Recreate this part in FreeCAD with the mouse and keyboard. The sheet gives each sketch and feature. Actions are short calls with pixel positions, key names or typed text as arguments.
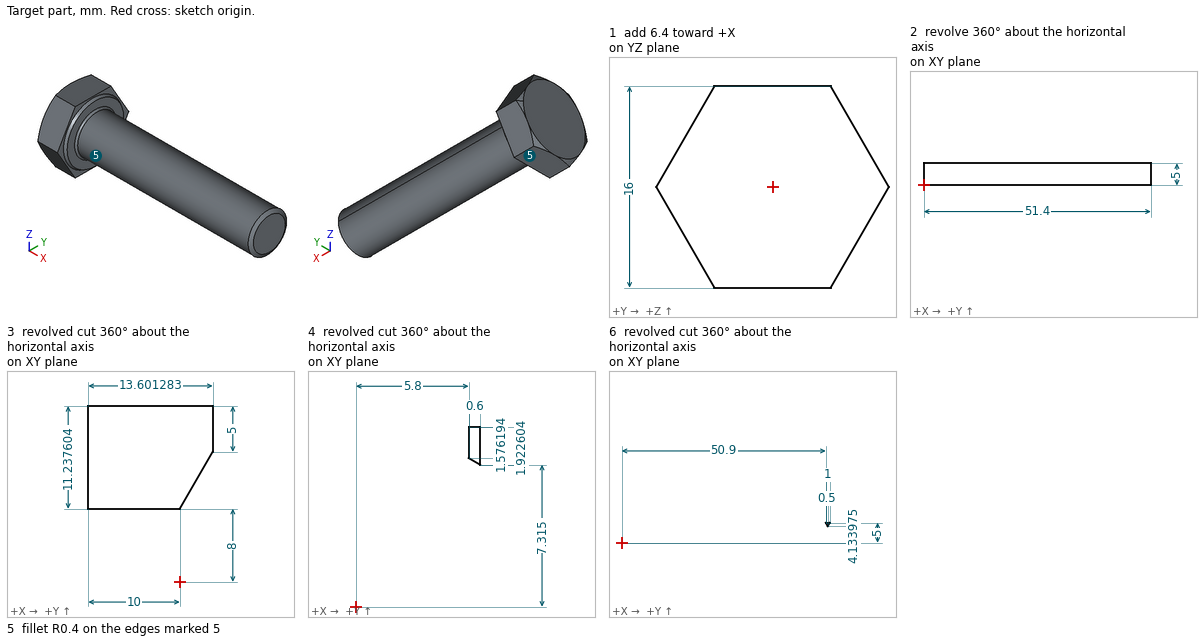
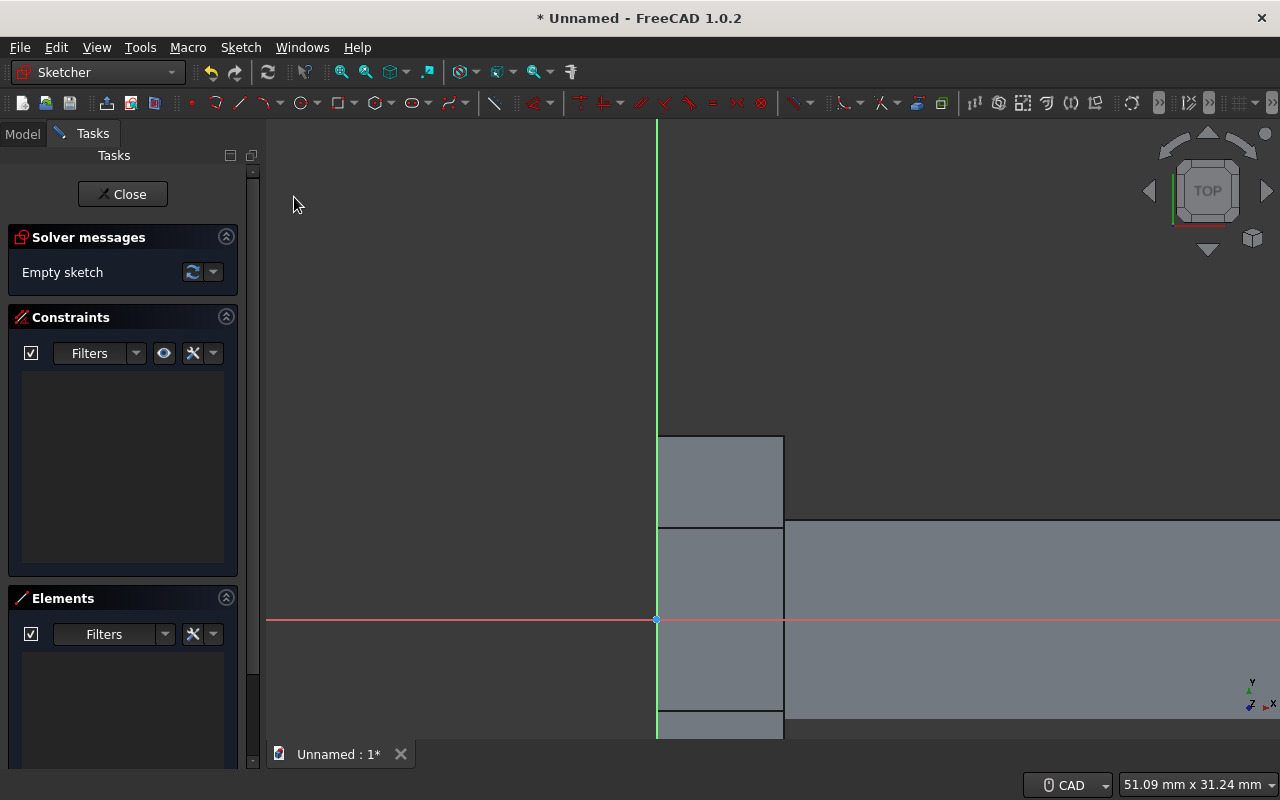
click(216, 104)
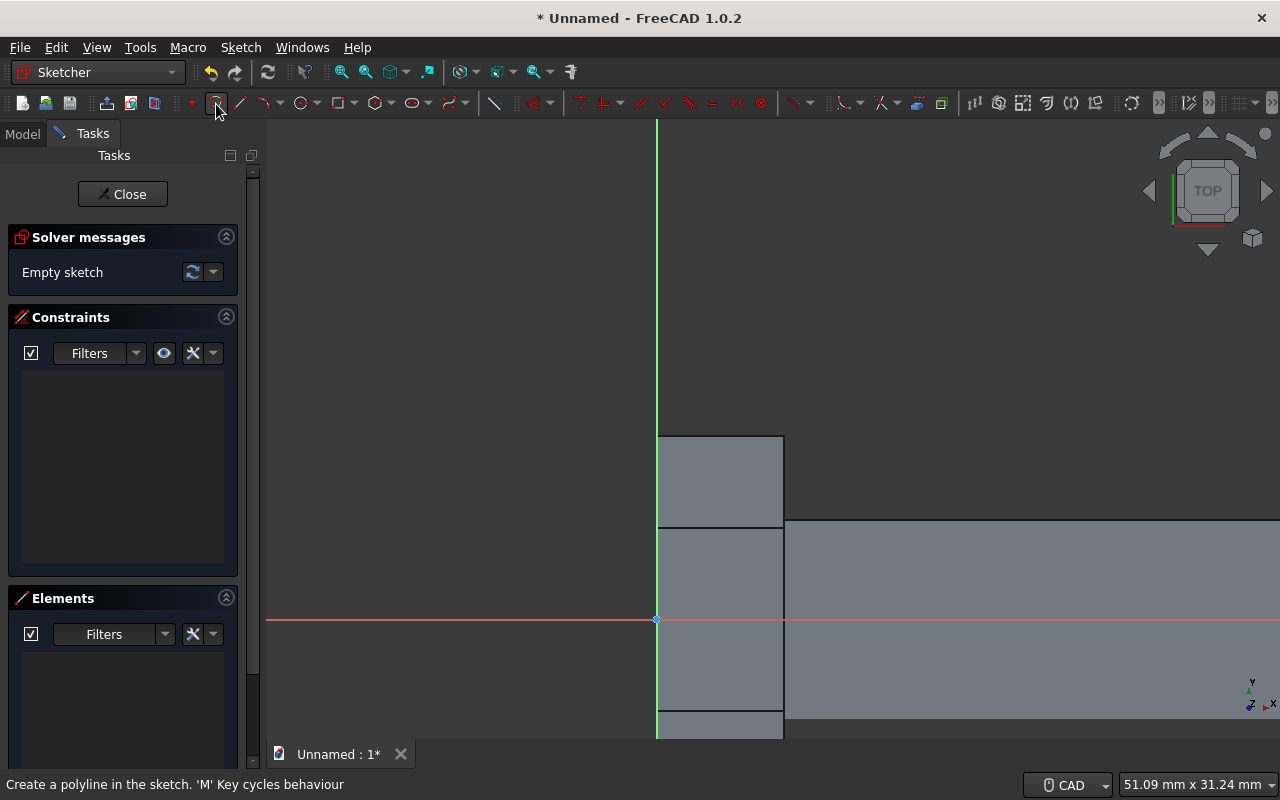
click(657, 461)
click(728, 337)
click(728, 238)
click(458, 238)
click(458, 461)
click(657, 462)
key(Escape)
key(Escape)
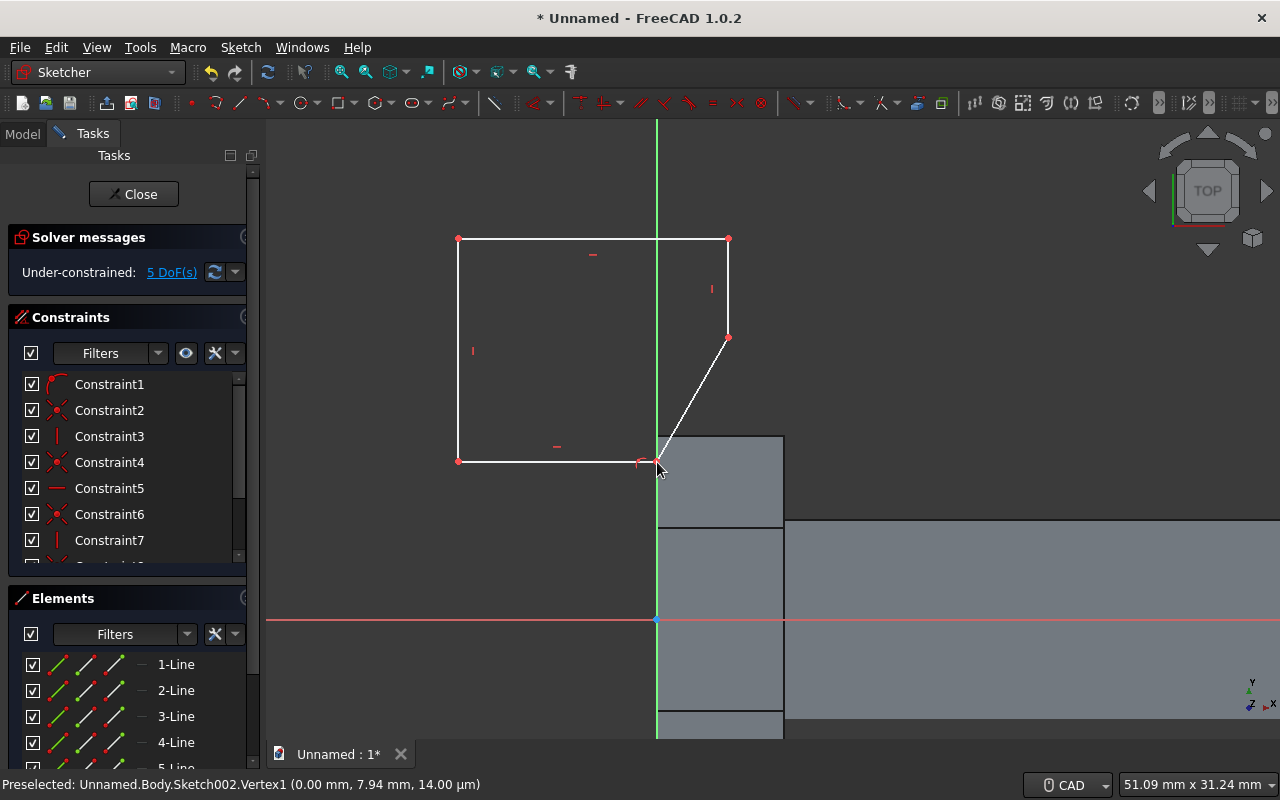
click(534, 104)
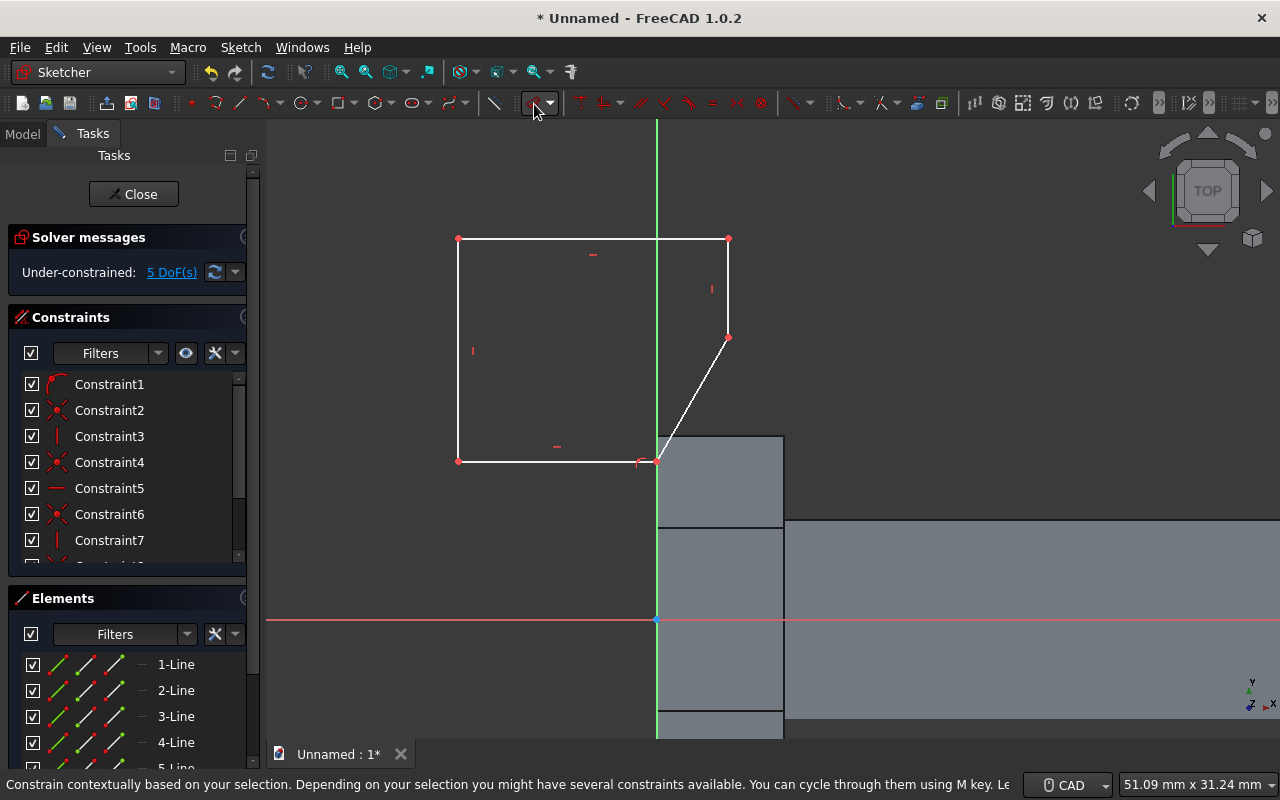
click(728, 308)
click(762, 288)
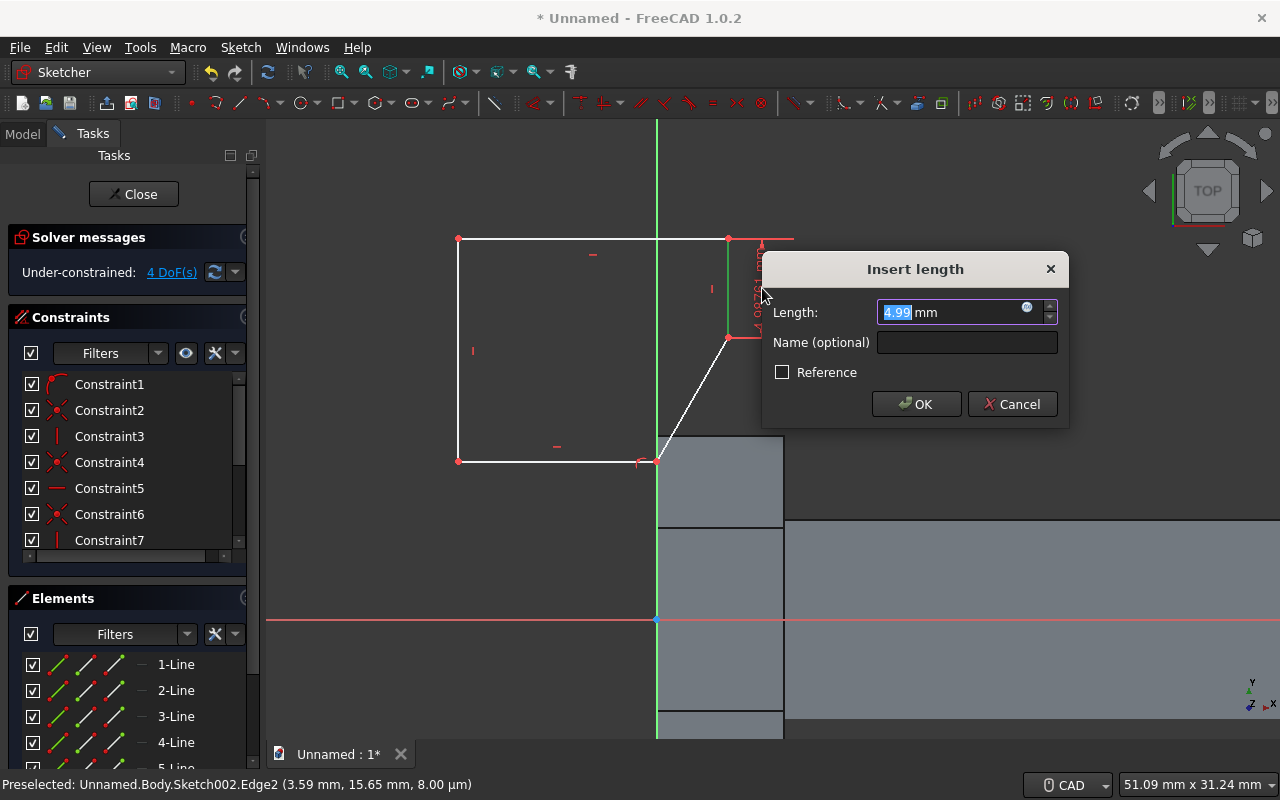
text(5)
key(Return)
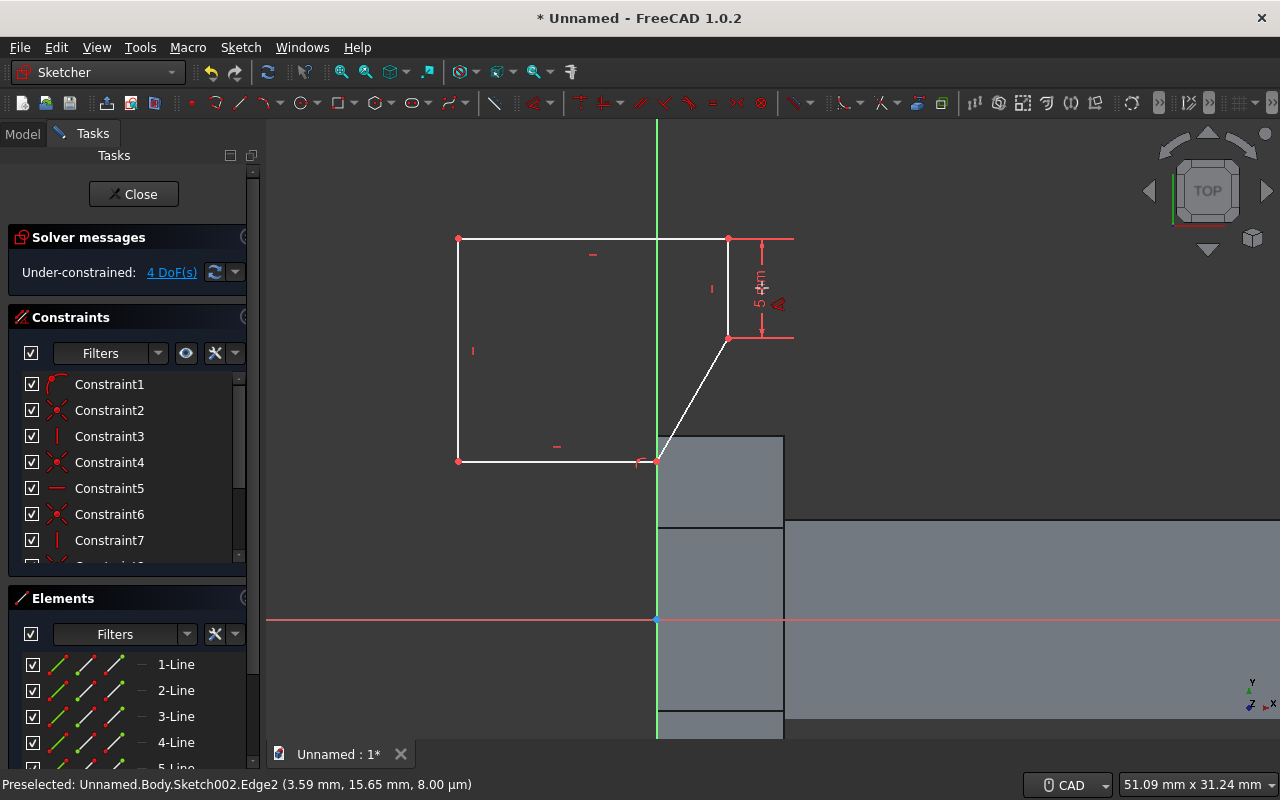
click(518, 462)
click(557, 496)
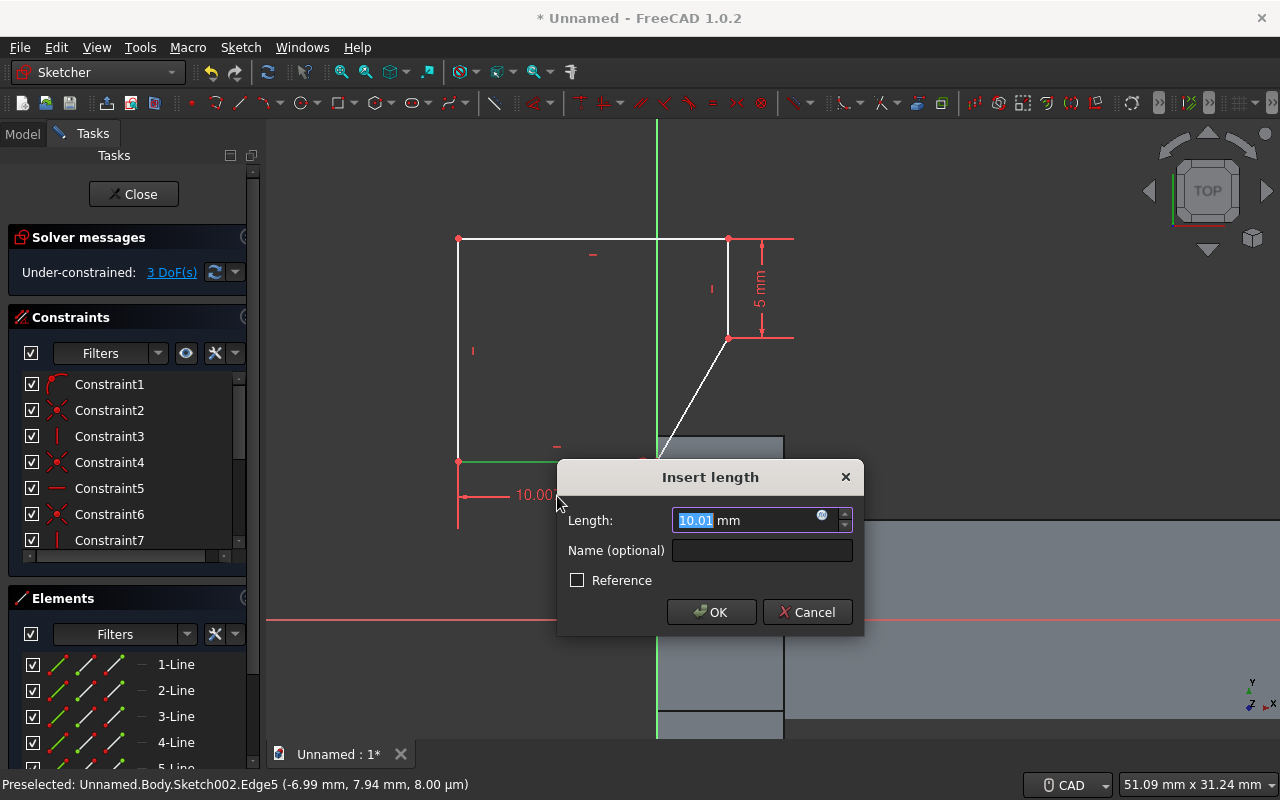
text(10)
key(Return)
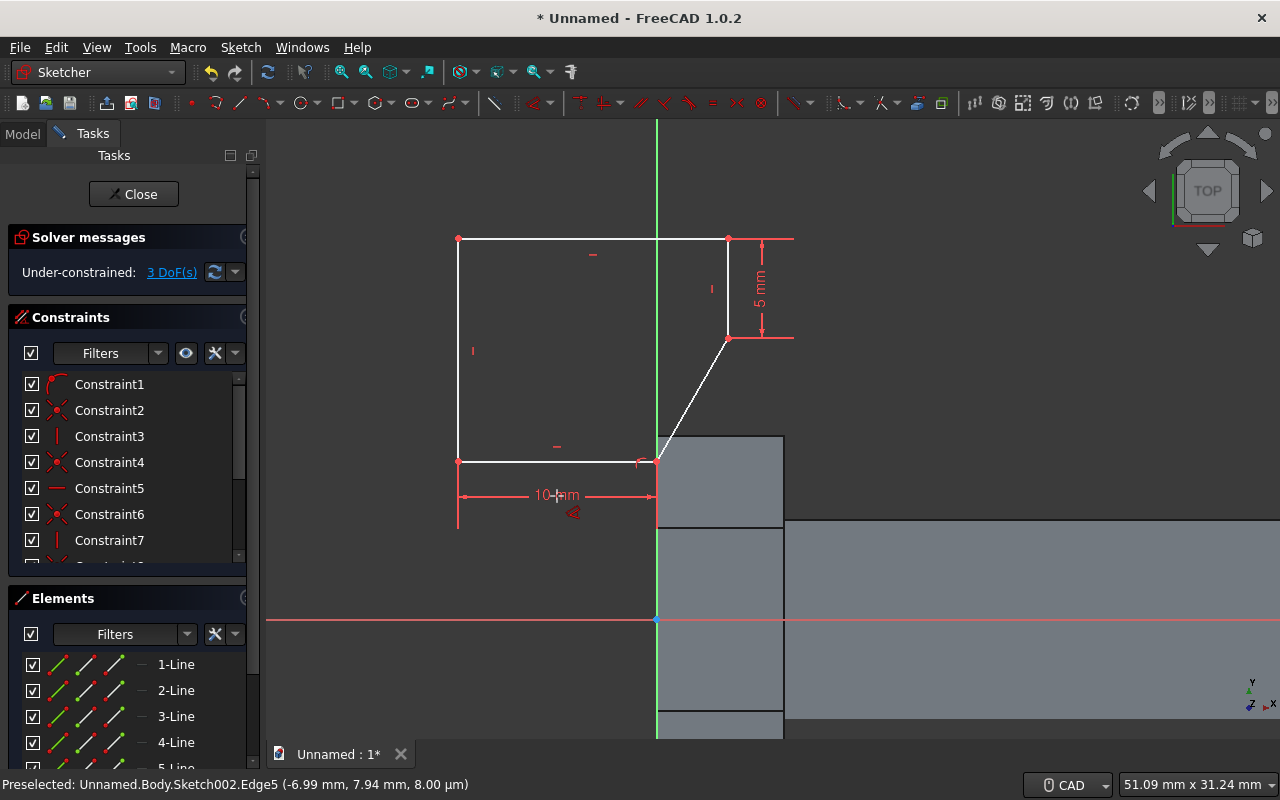
click(657, 462)
click(691, 541)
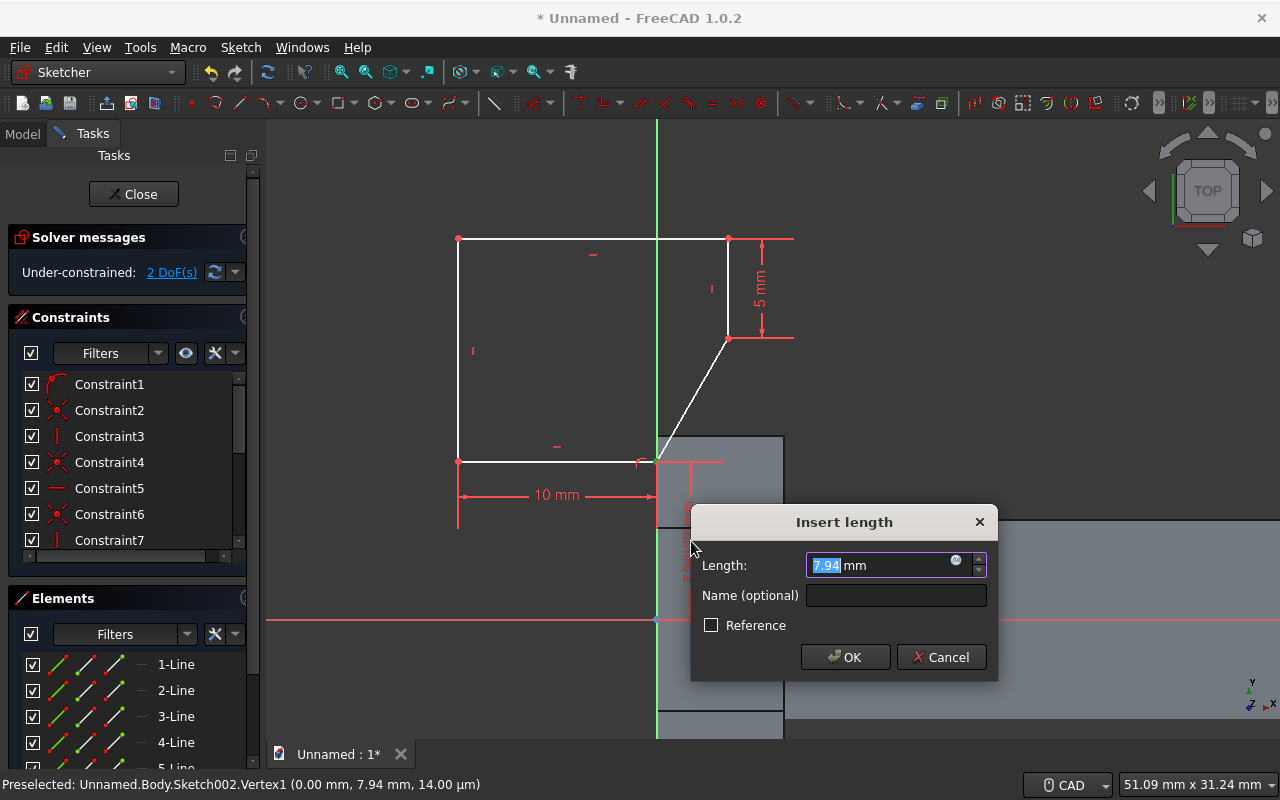
text(8)
key(Return)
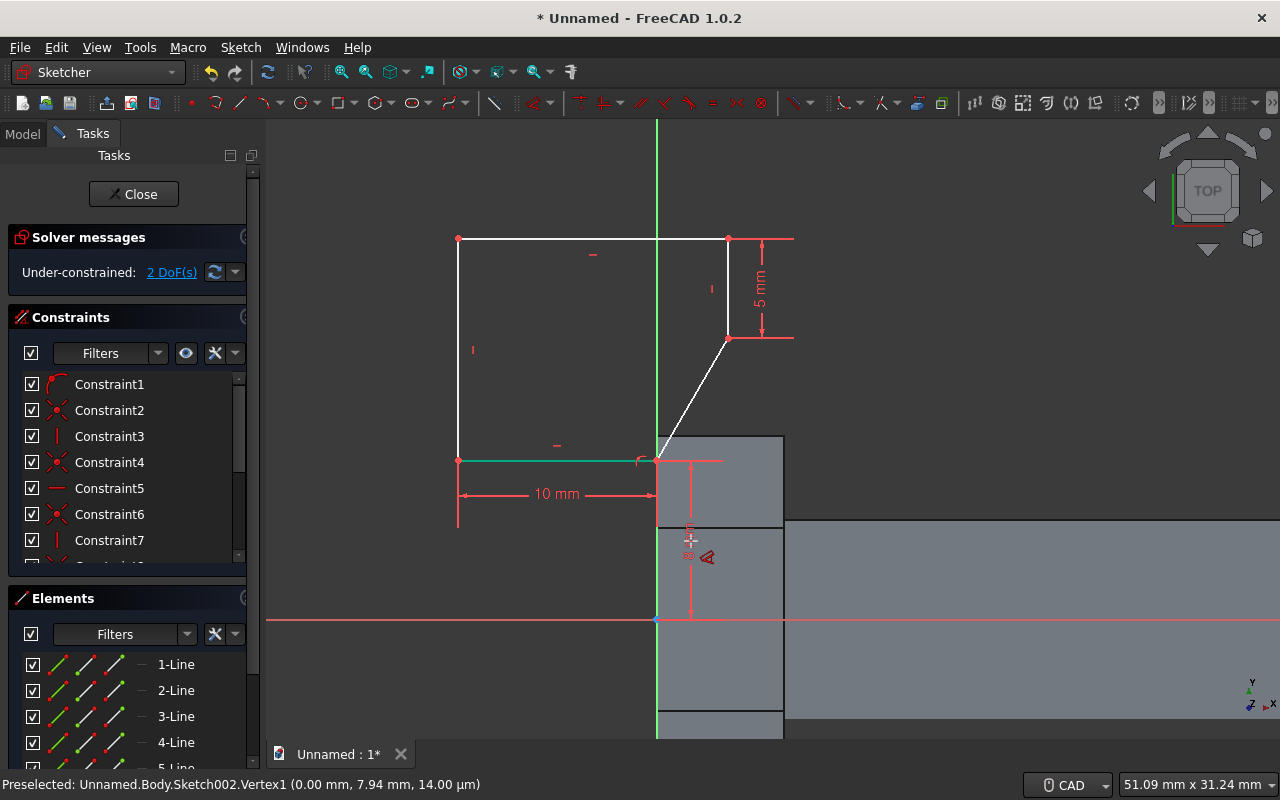
scroll(647, 239, up, 2)